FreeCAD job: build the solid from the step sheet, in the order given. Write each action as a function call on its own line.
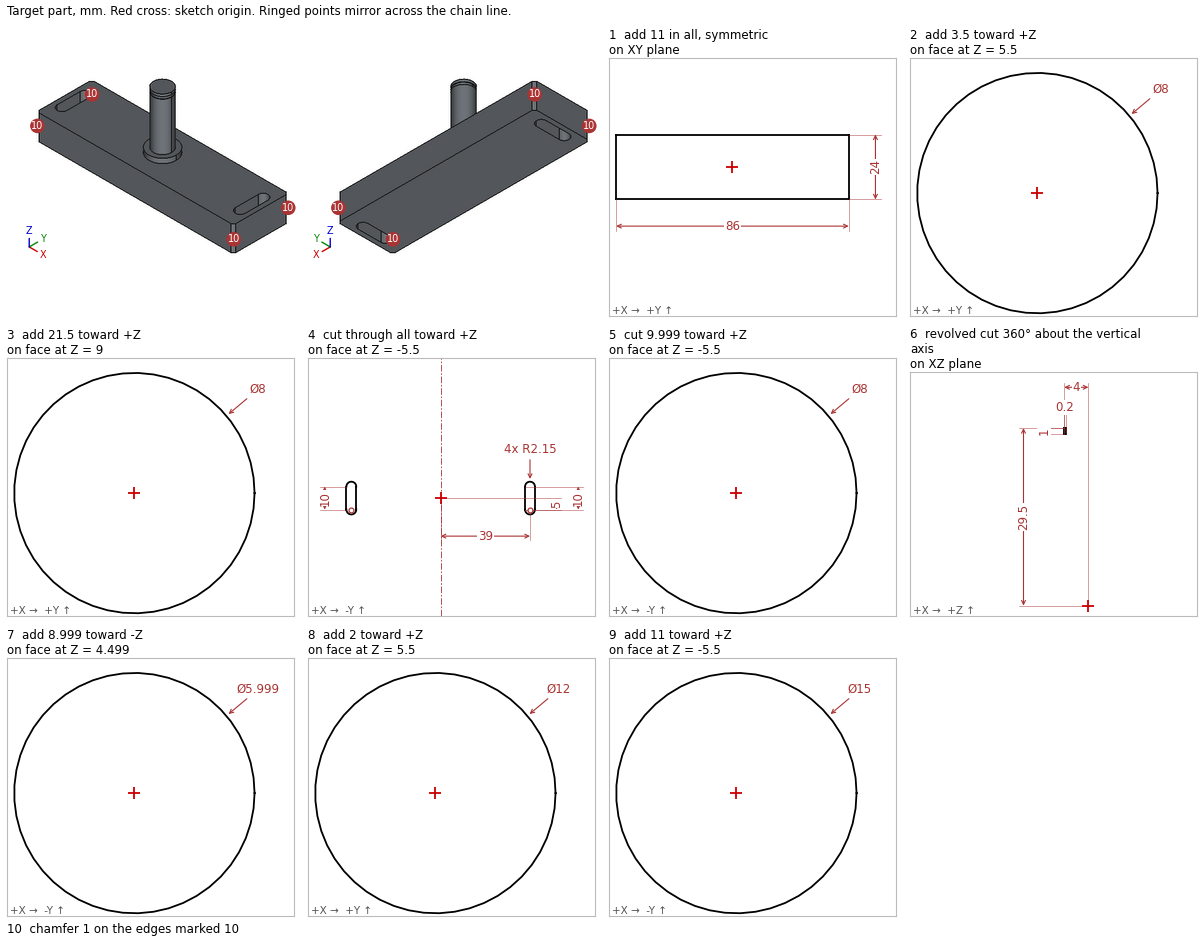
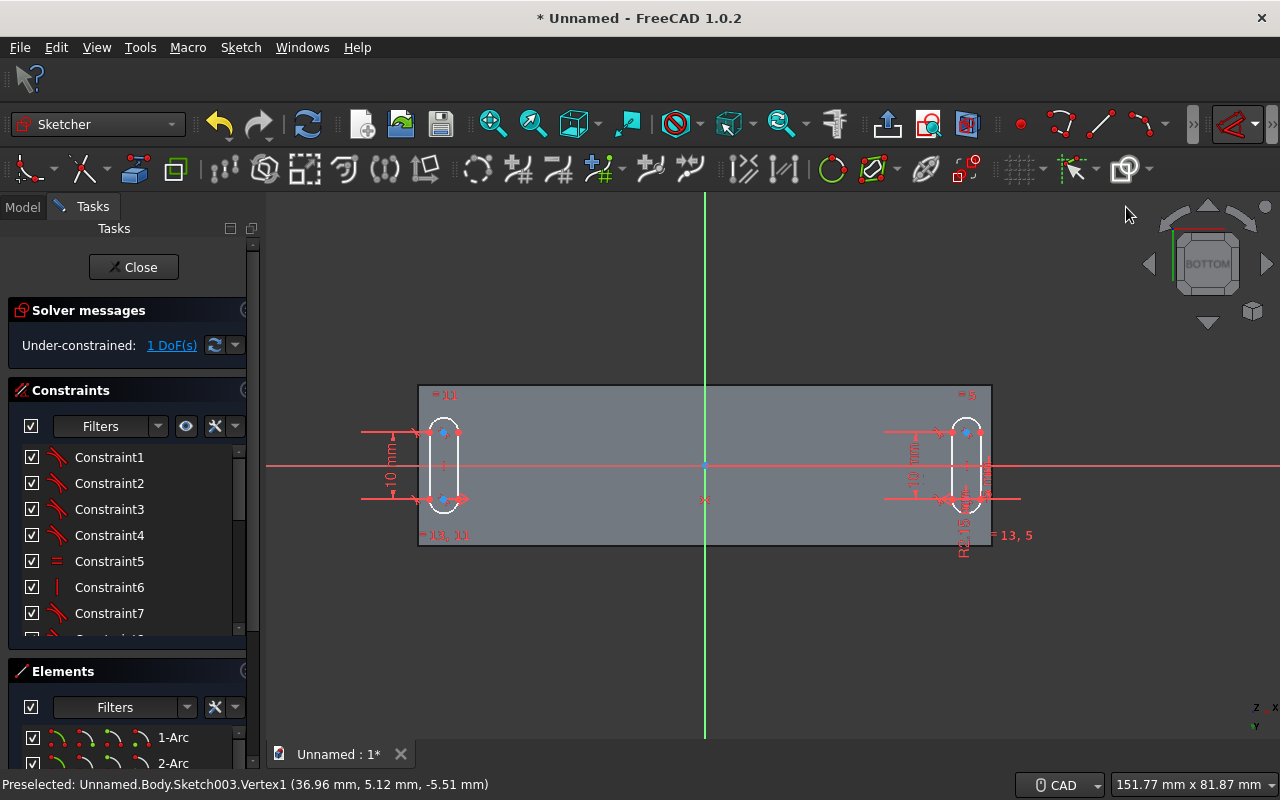
click(966, 499)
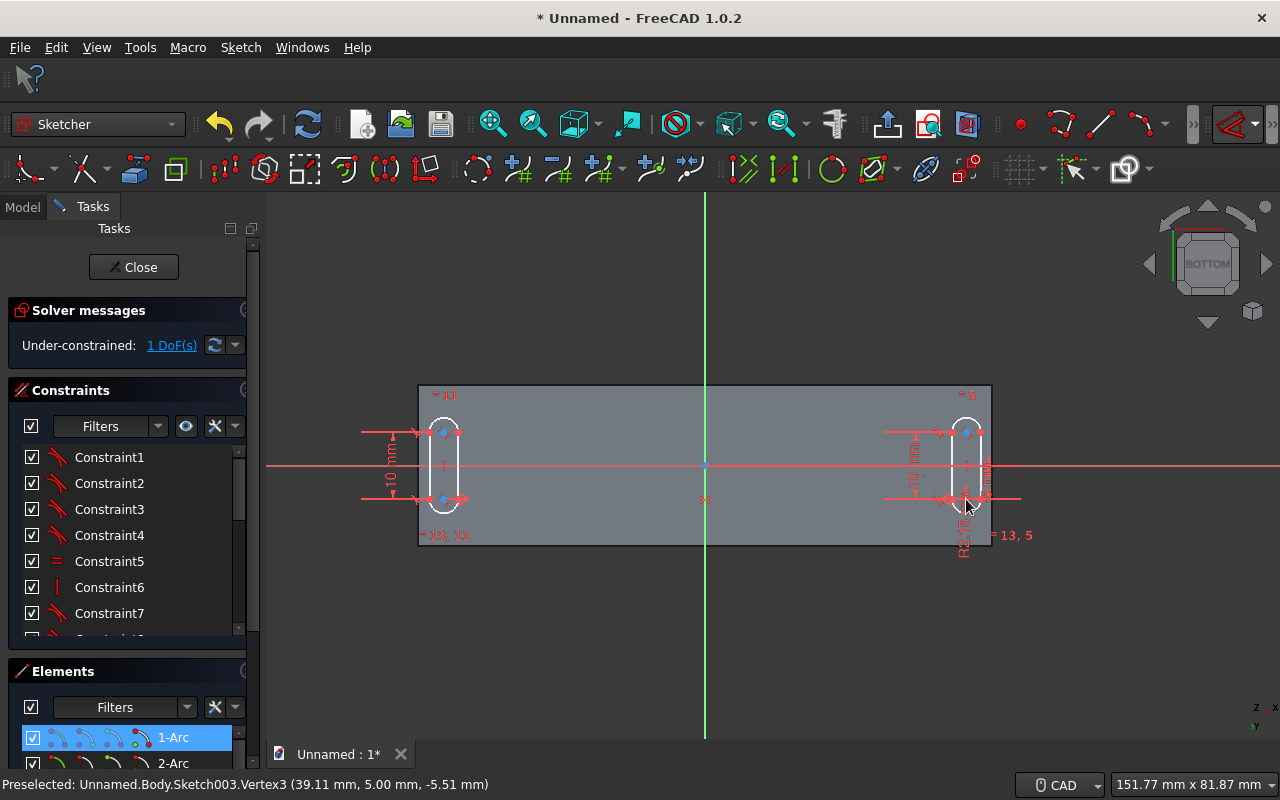
click(1258, 124)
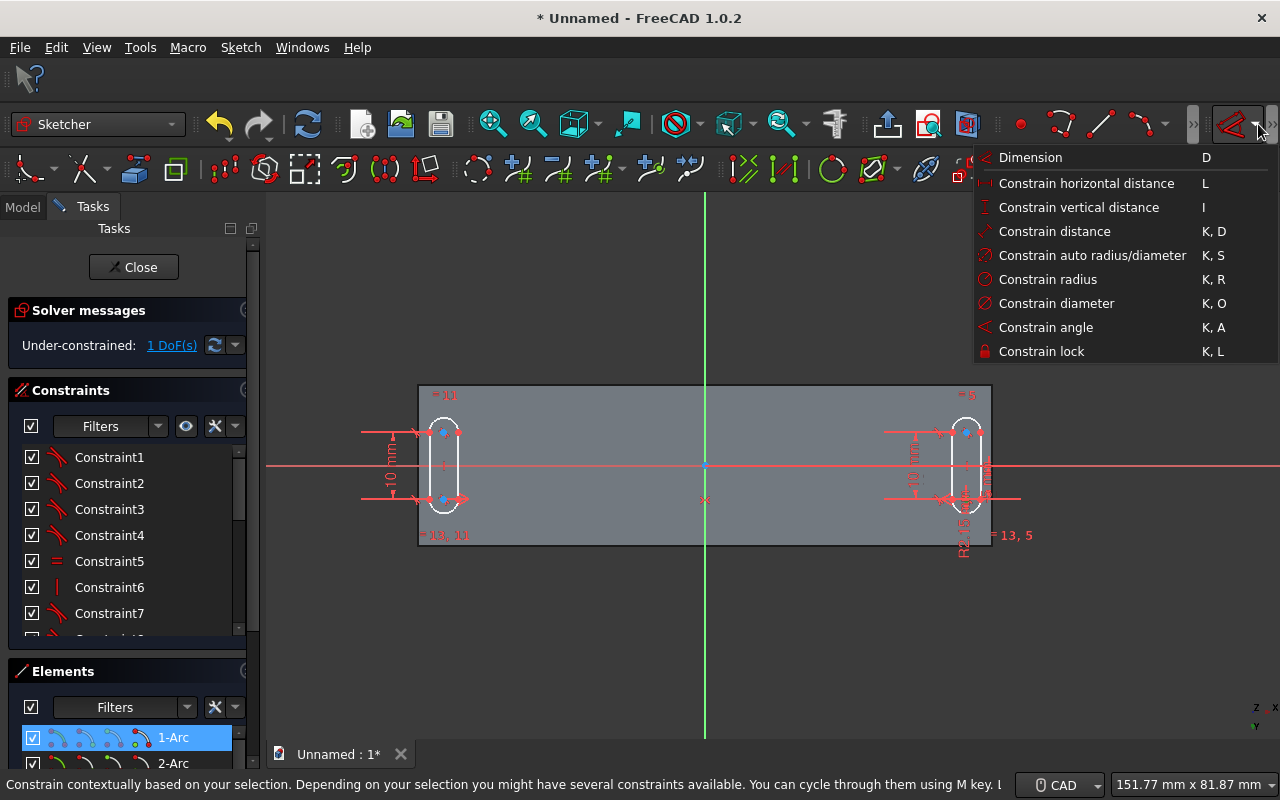
click(1126, 183)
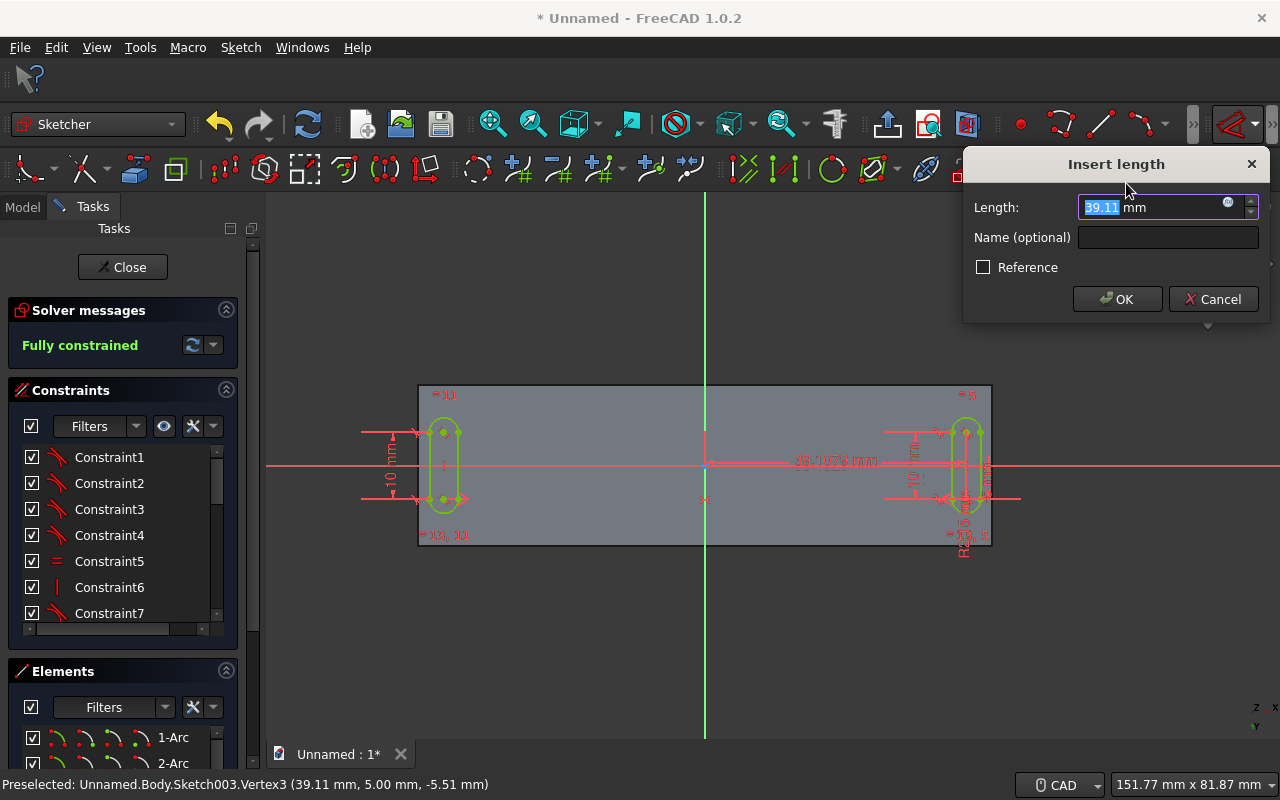
text(39)
key(Return)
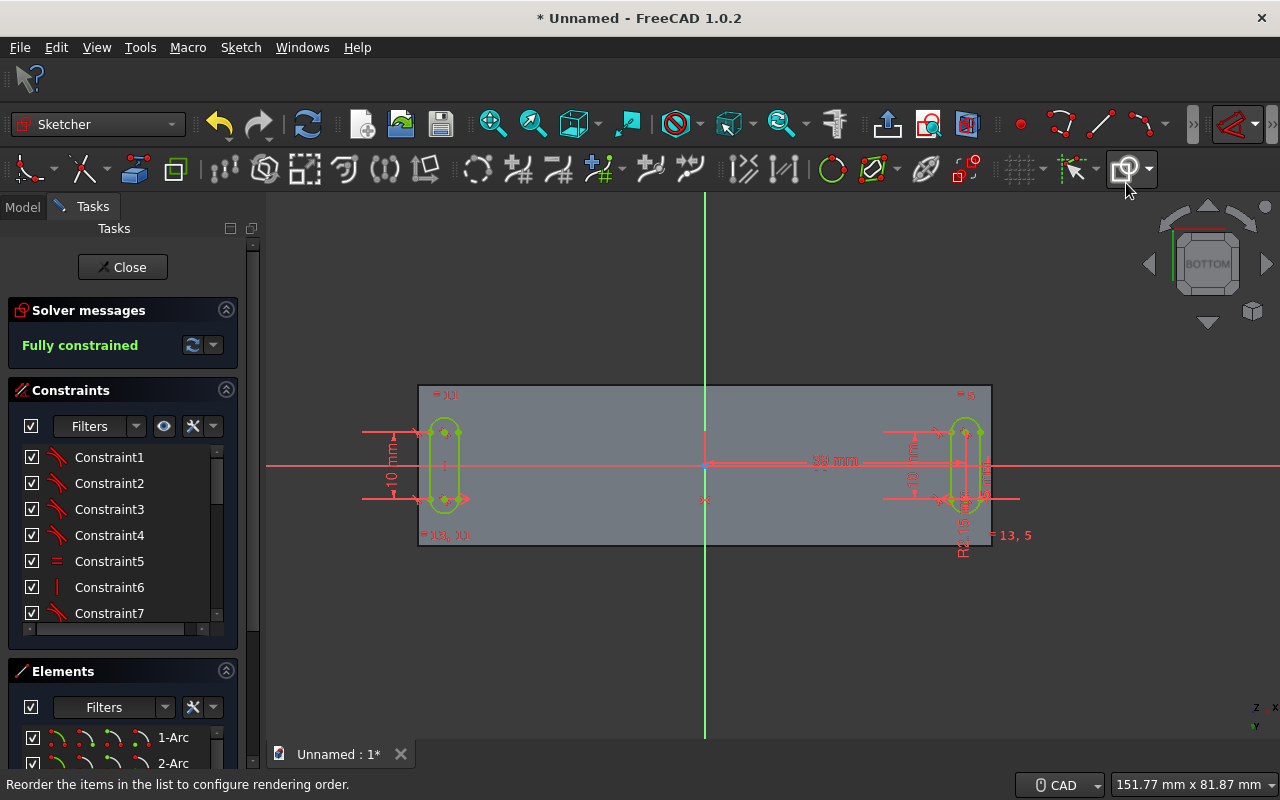
click(123, 267)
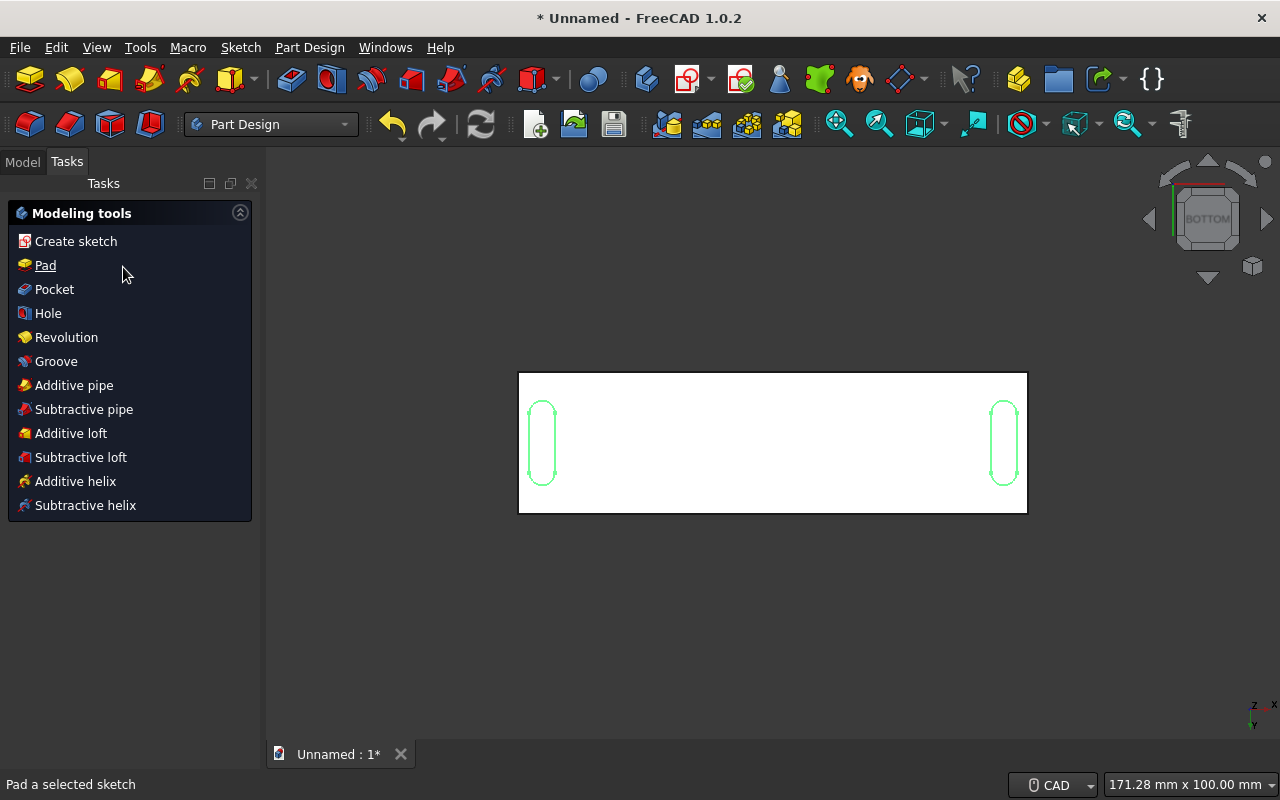
click(292, 80)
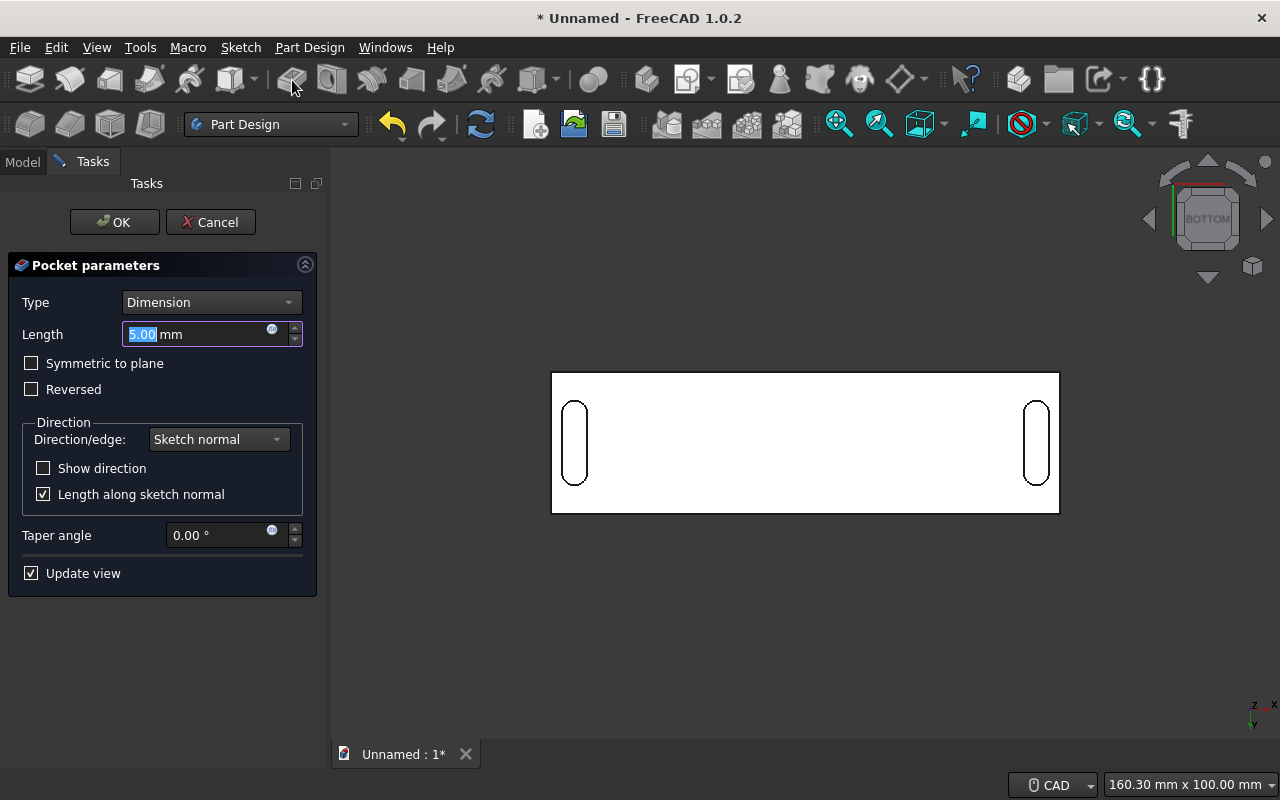
click(212, 302)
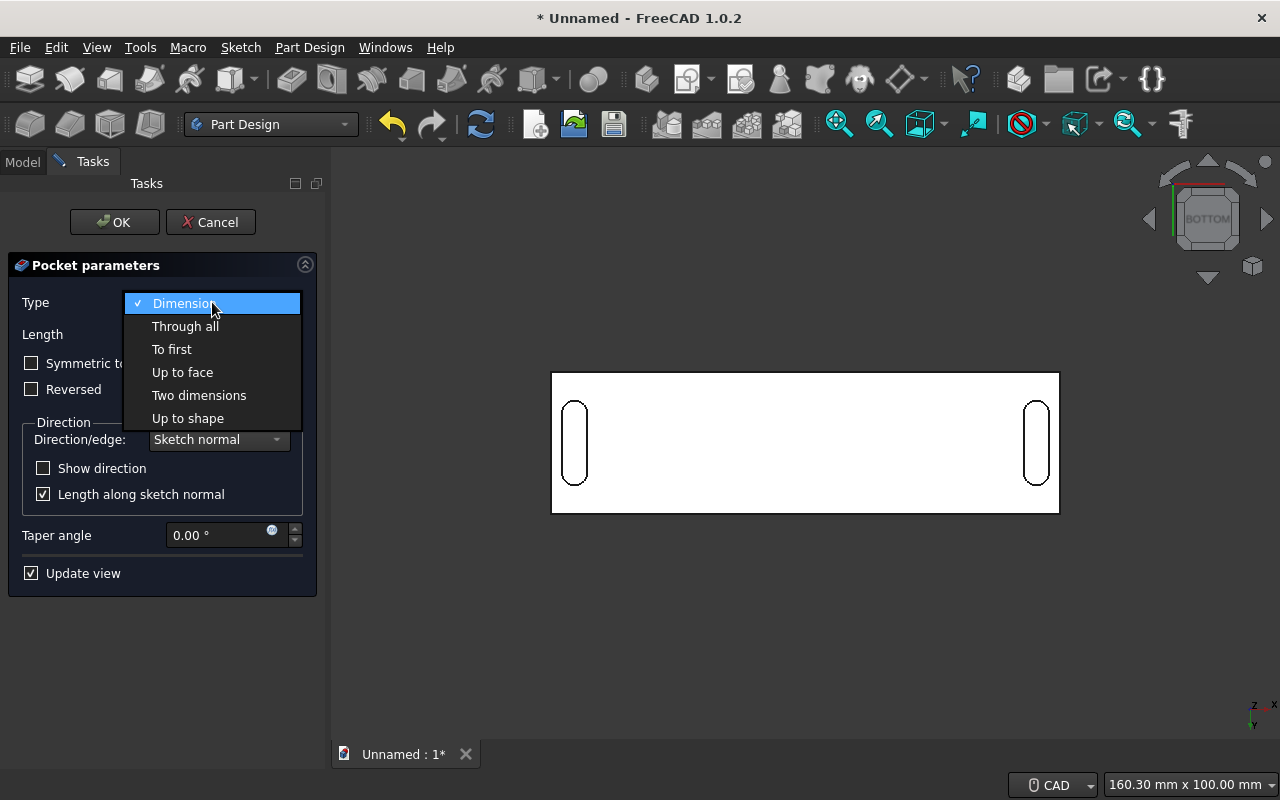
click(212, 326)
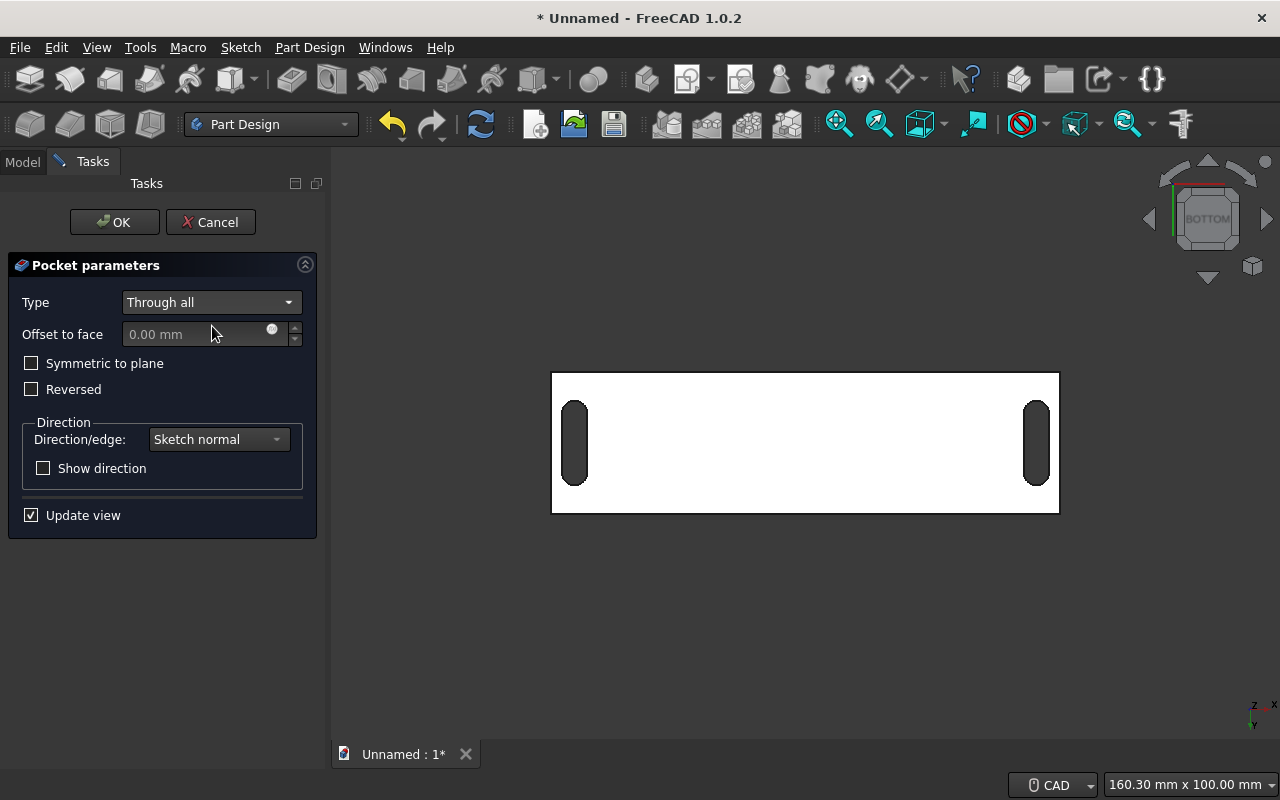
click(115, 222)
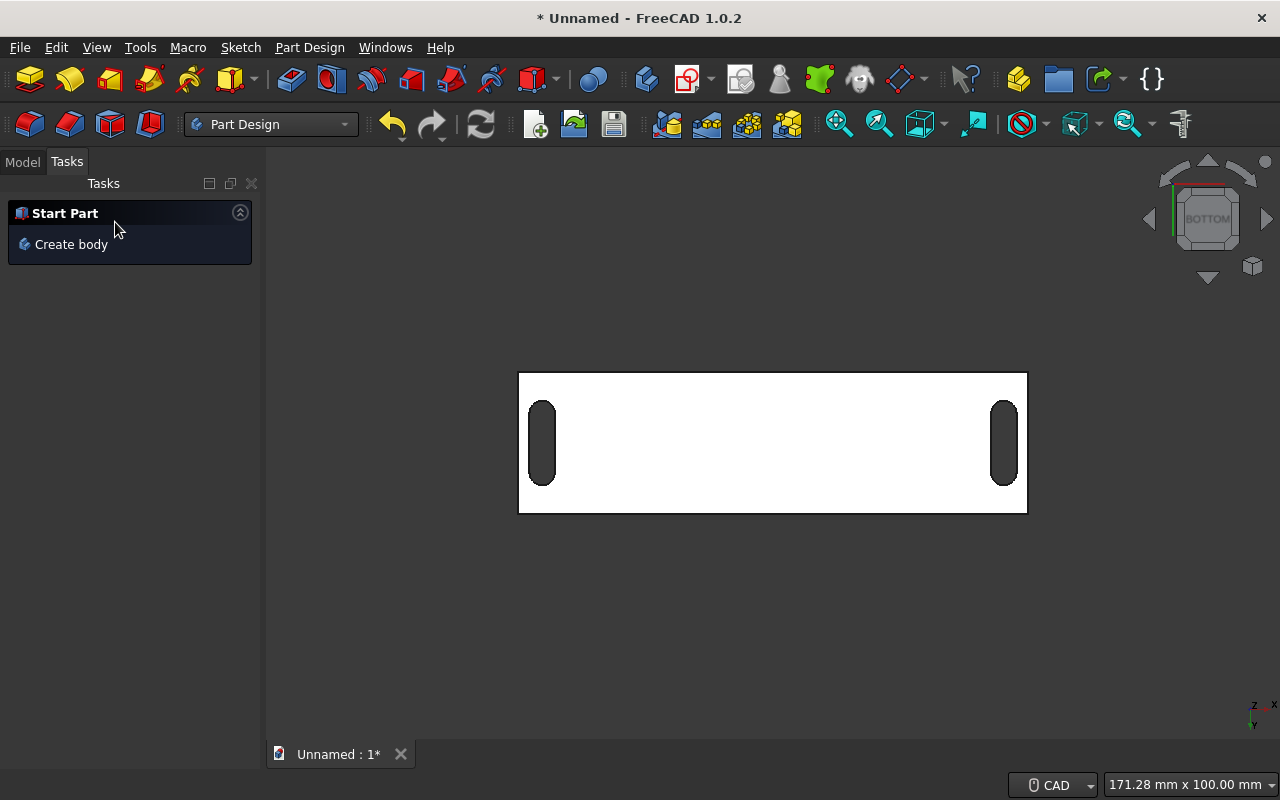
click(918, 442)